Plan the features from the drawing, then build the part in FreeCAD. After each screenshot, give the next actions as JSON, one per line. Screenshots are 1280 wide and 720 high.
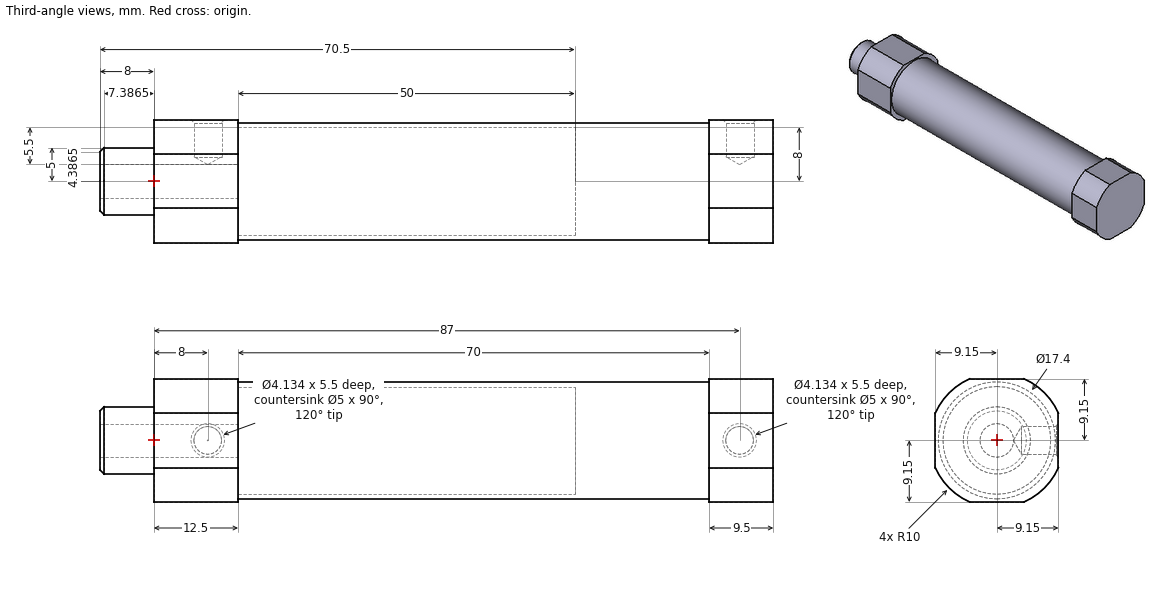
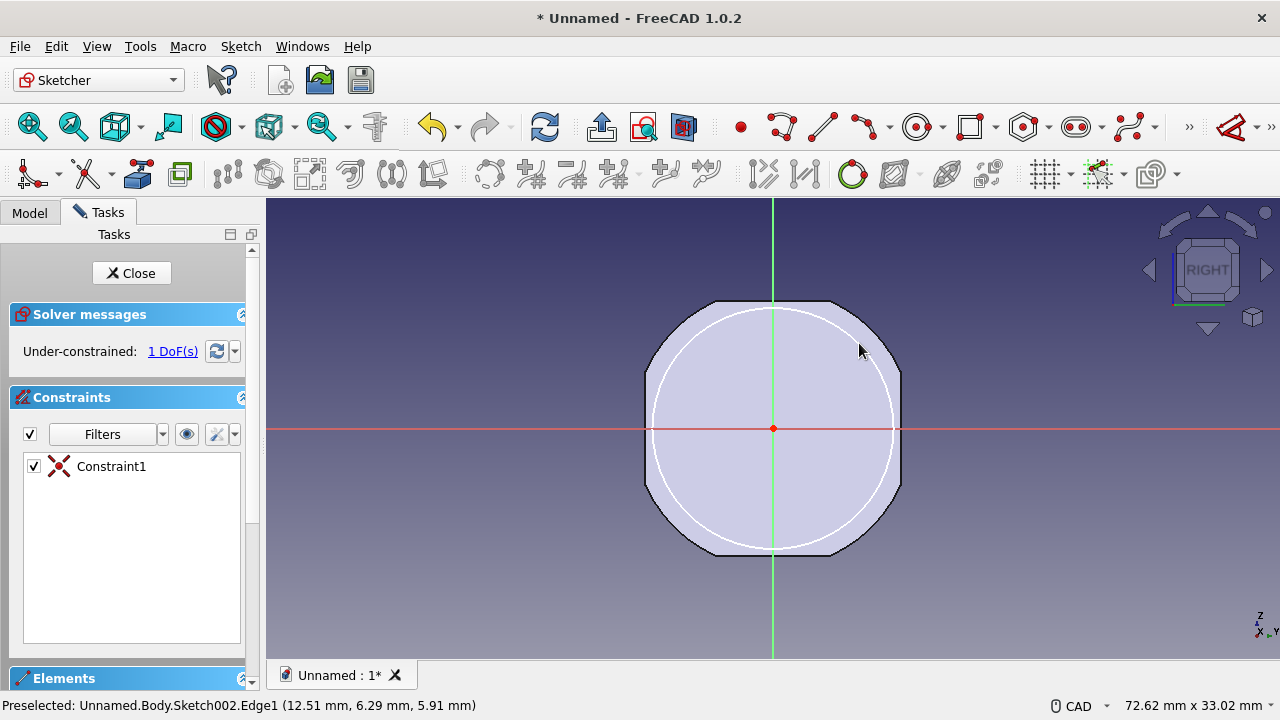
{"action": "left_click", "coordinate": [1230, 128]}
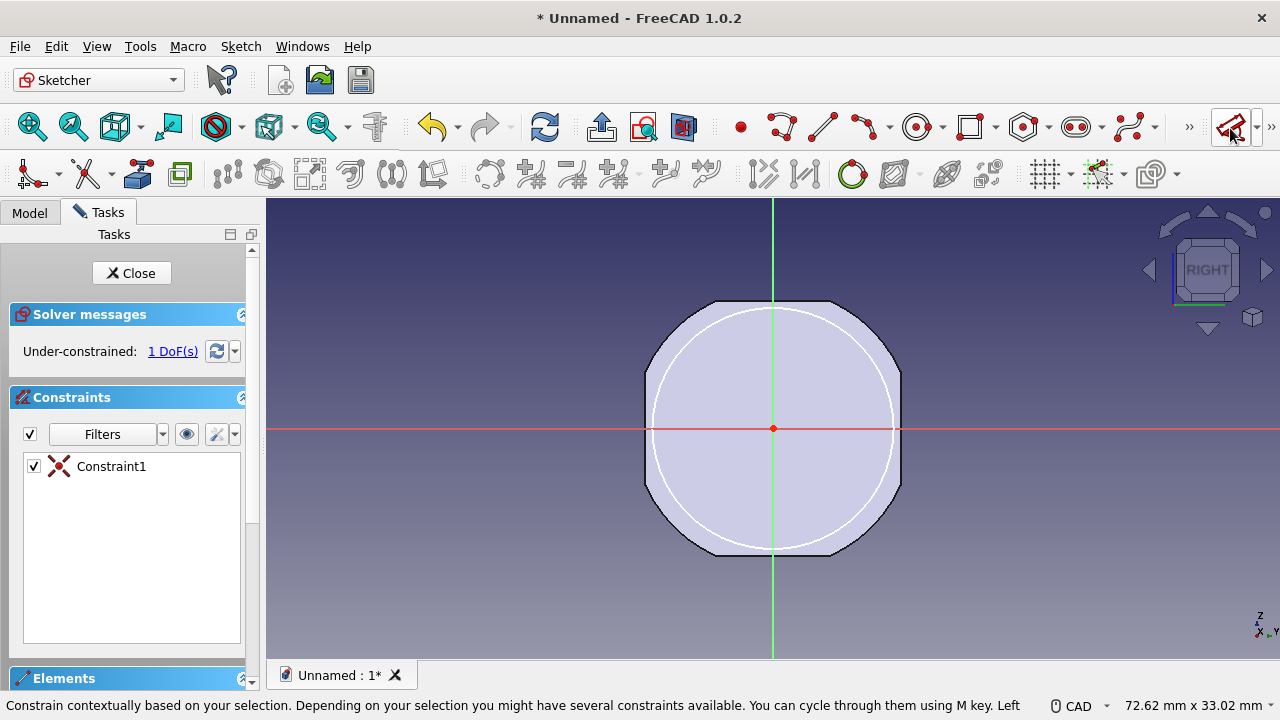
{"action": "left_click", "coordinate": [858, 343]}
{"action": "left_click", "coordinate": [881, 320]}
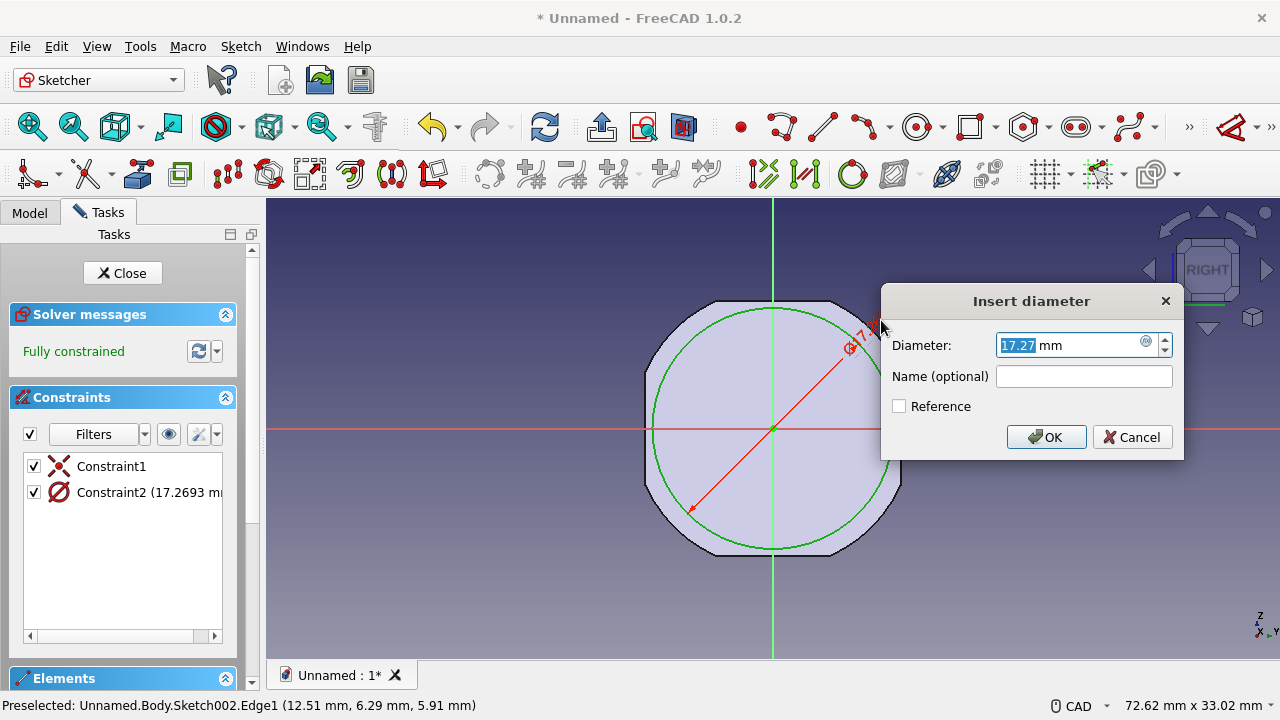
{"action": "type", "text": "17.4"}
{"action": "key", "text": "Return"}
{"action": "key", "text": "Escape"}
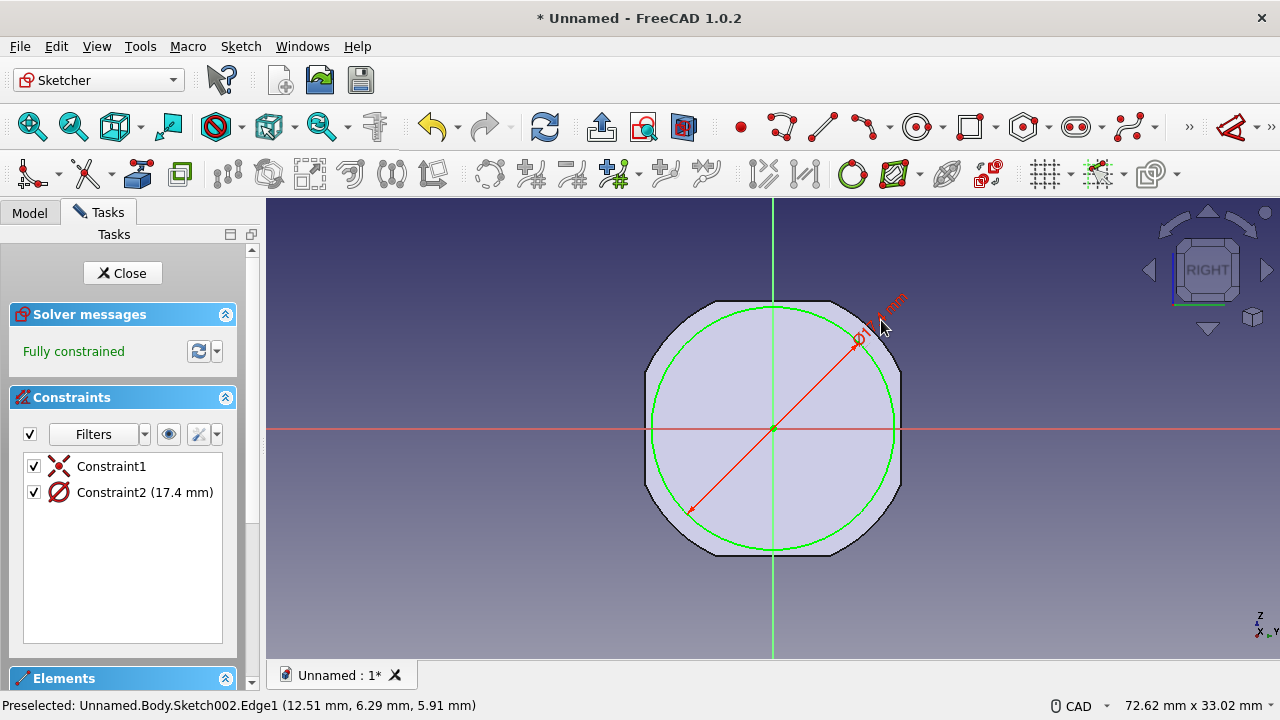
{"action": "left_click", "coordinate": [123, 273]}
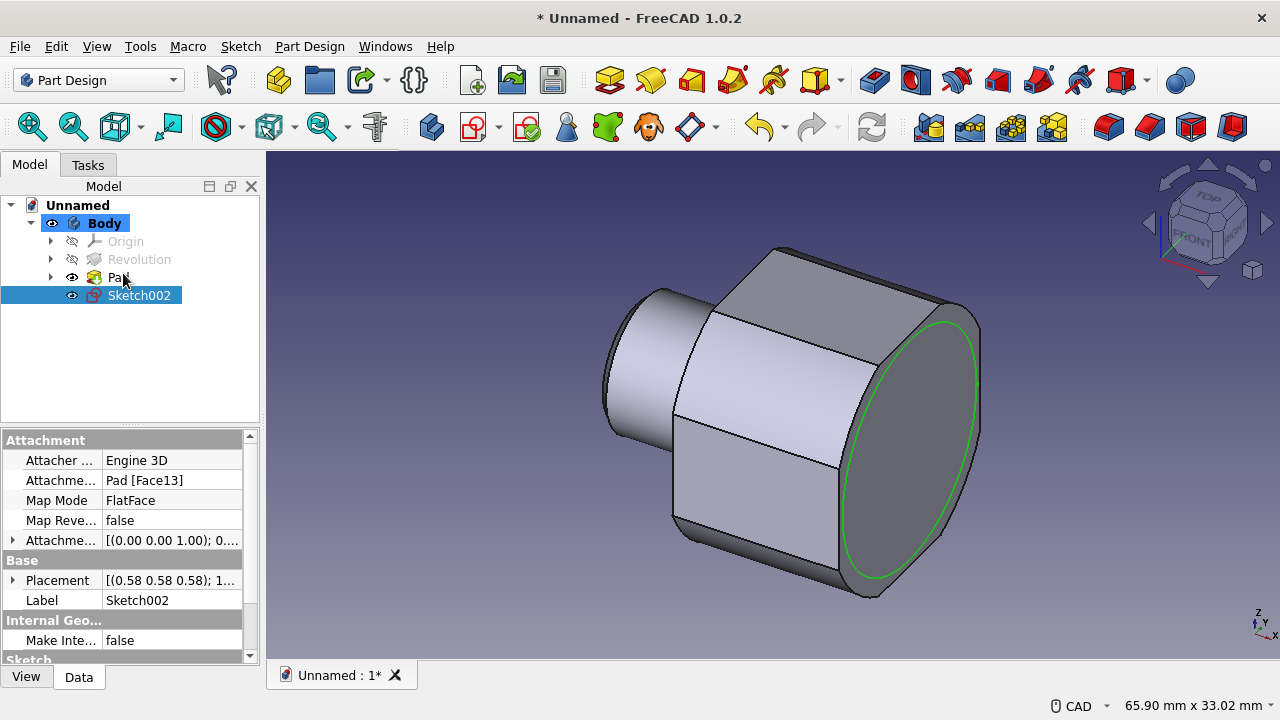
{"action": "left_click", "coordinate": [610, 80]}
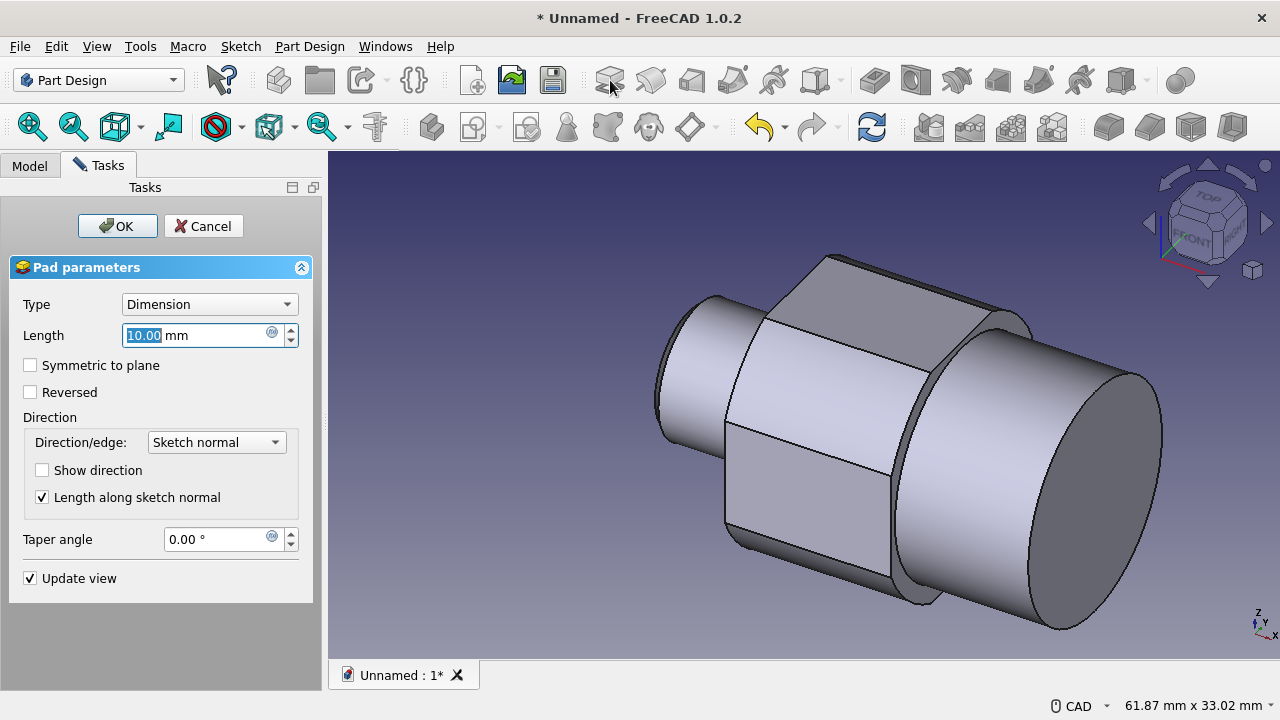
{"action": "type", "text": "70"}
{"action": "key", "text": "Tab"}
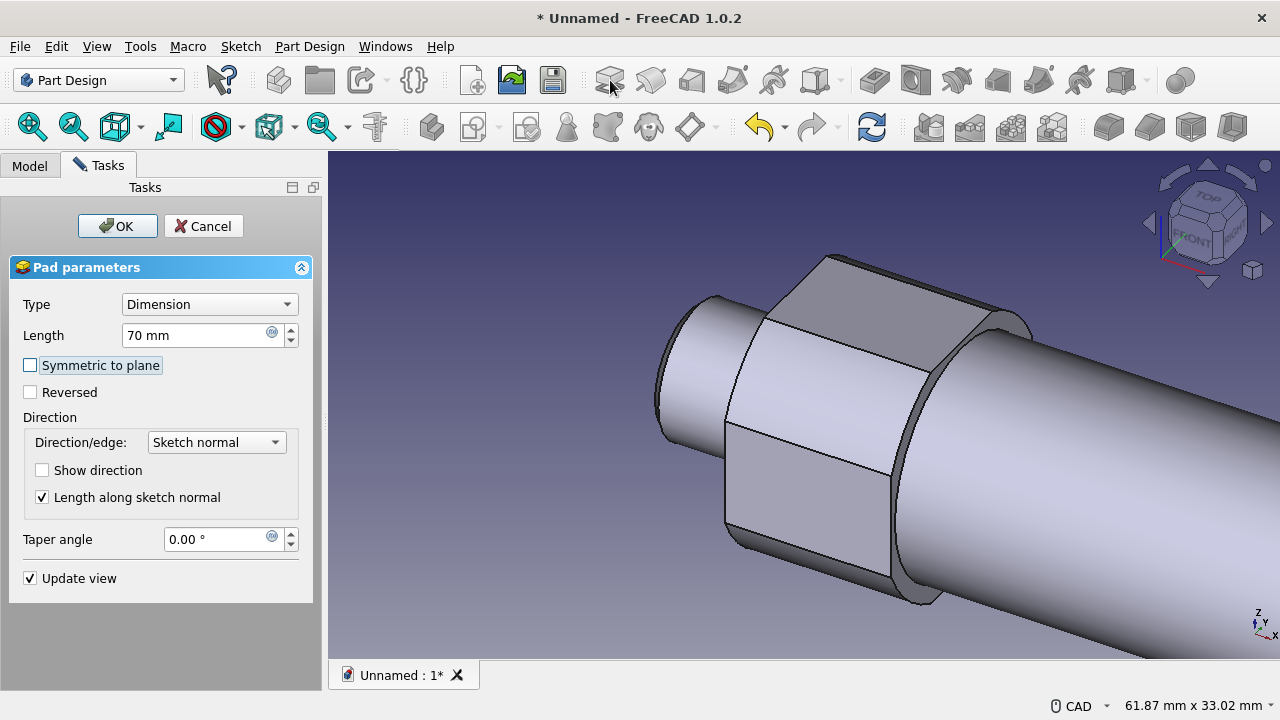
{"action": "left_click", "coordinate": [118, 226]}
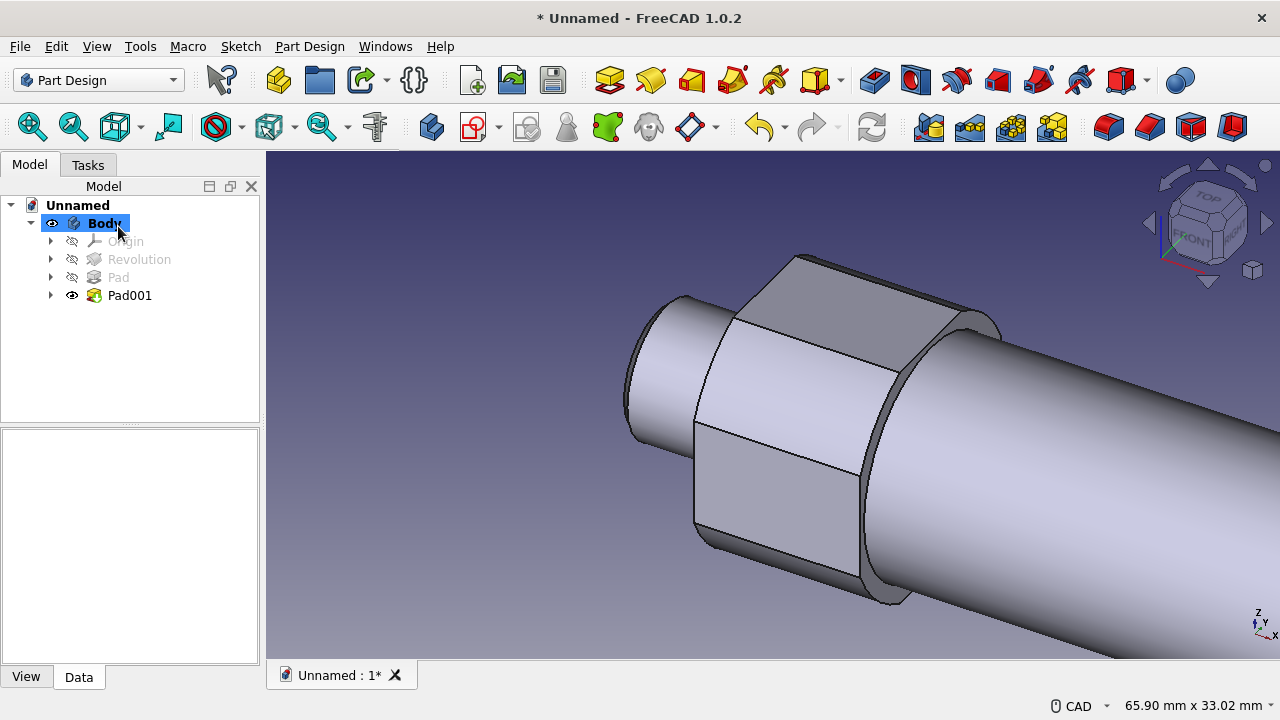
{"action": "left_click", "coordinate": [33, 128]}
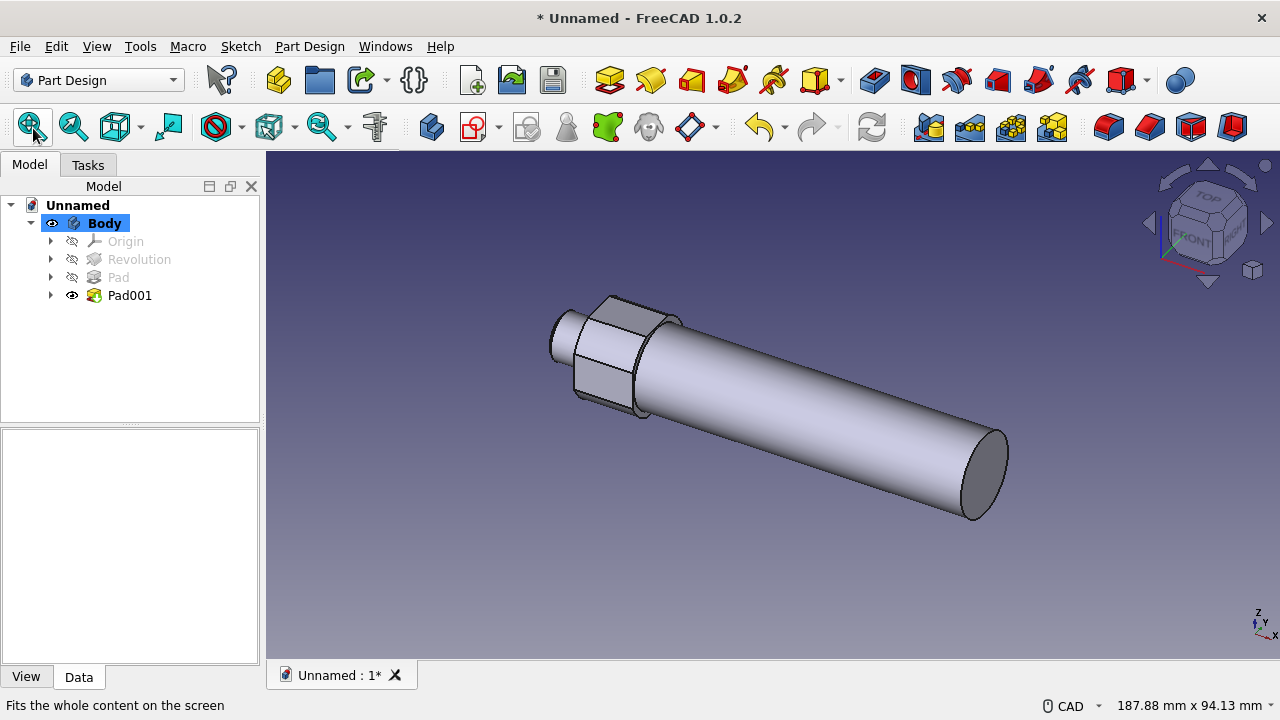
{"action": "left_click", "coordinate": [984, 474]}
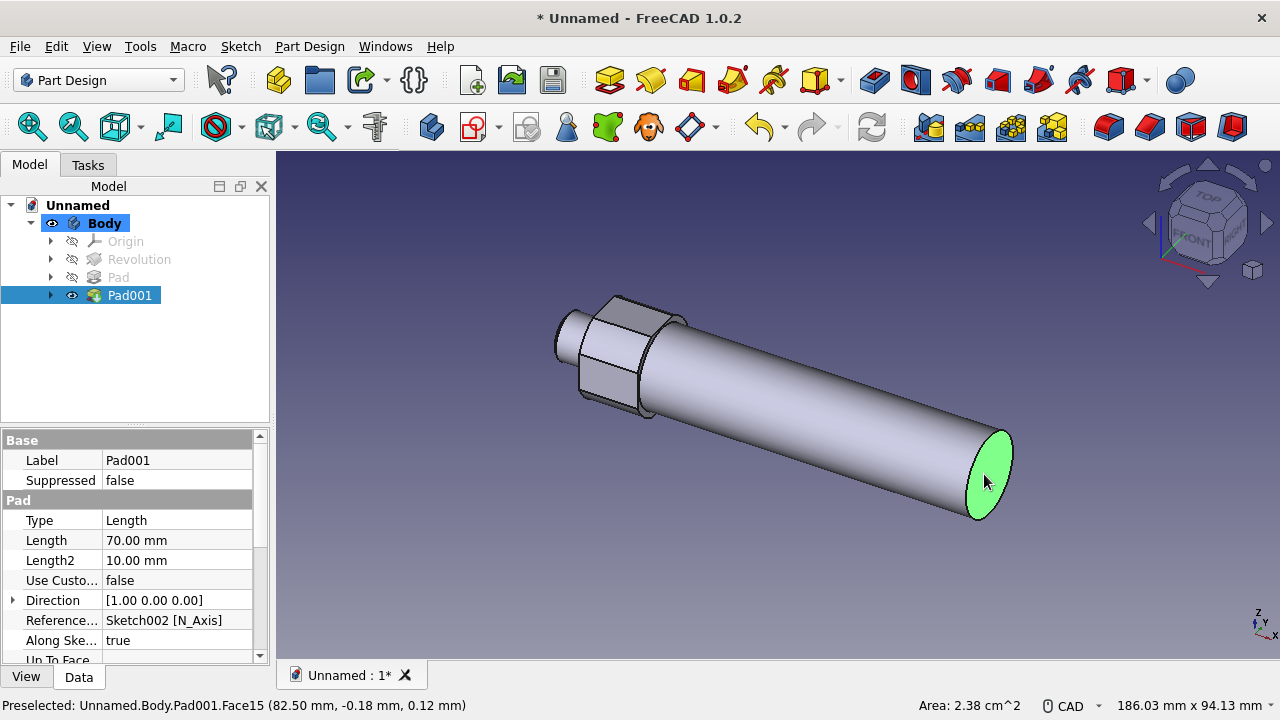
{"action": "left_click", "coordinate": [472, 128]}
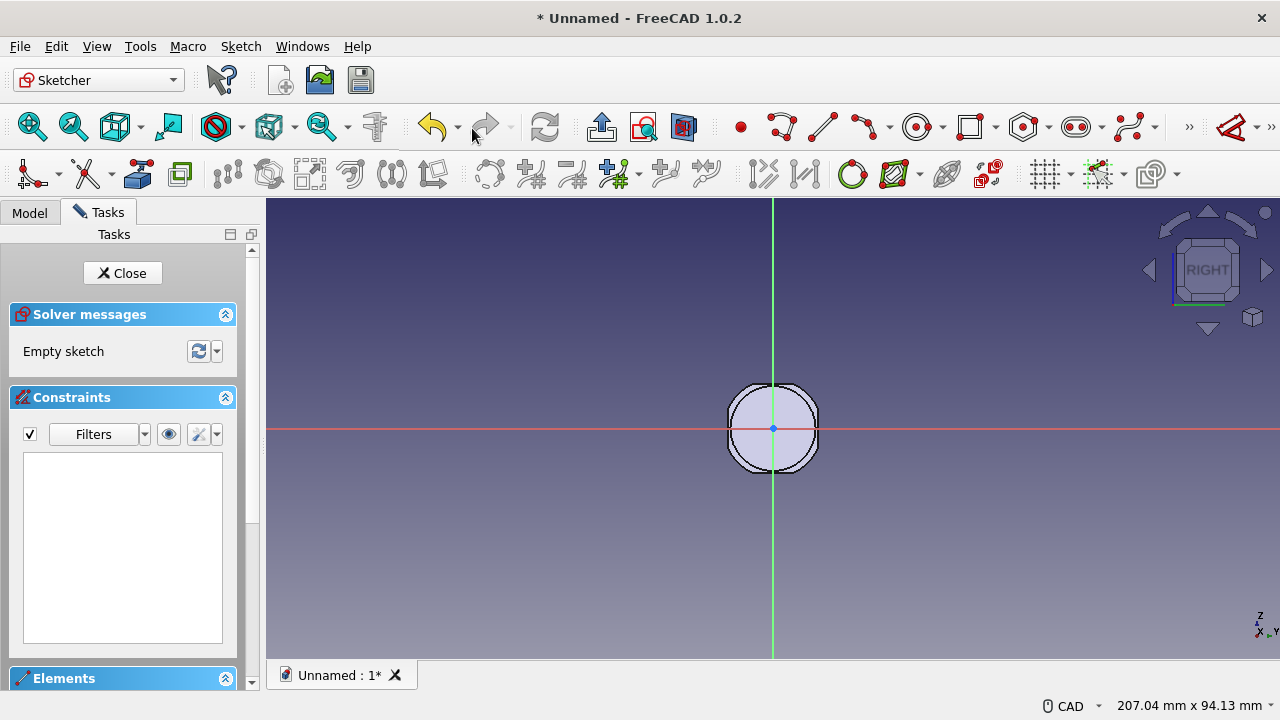
{"action": "scroll", "coordinate": [803, 428], "scroll_direction": "up", "scroll_amount": 6}